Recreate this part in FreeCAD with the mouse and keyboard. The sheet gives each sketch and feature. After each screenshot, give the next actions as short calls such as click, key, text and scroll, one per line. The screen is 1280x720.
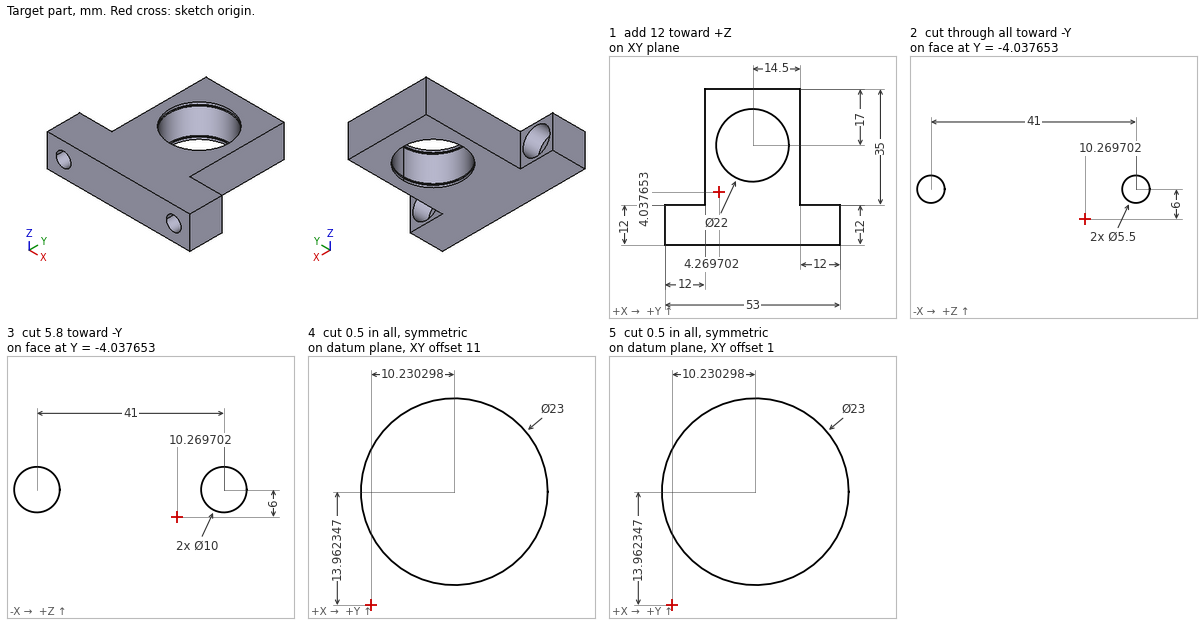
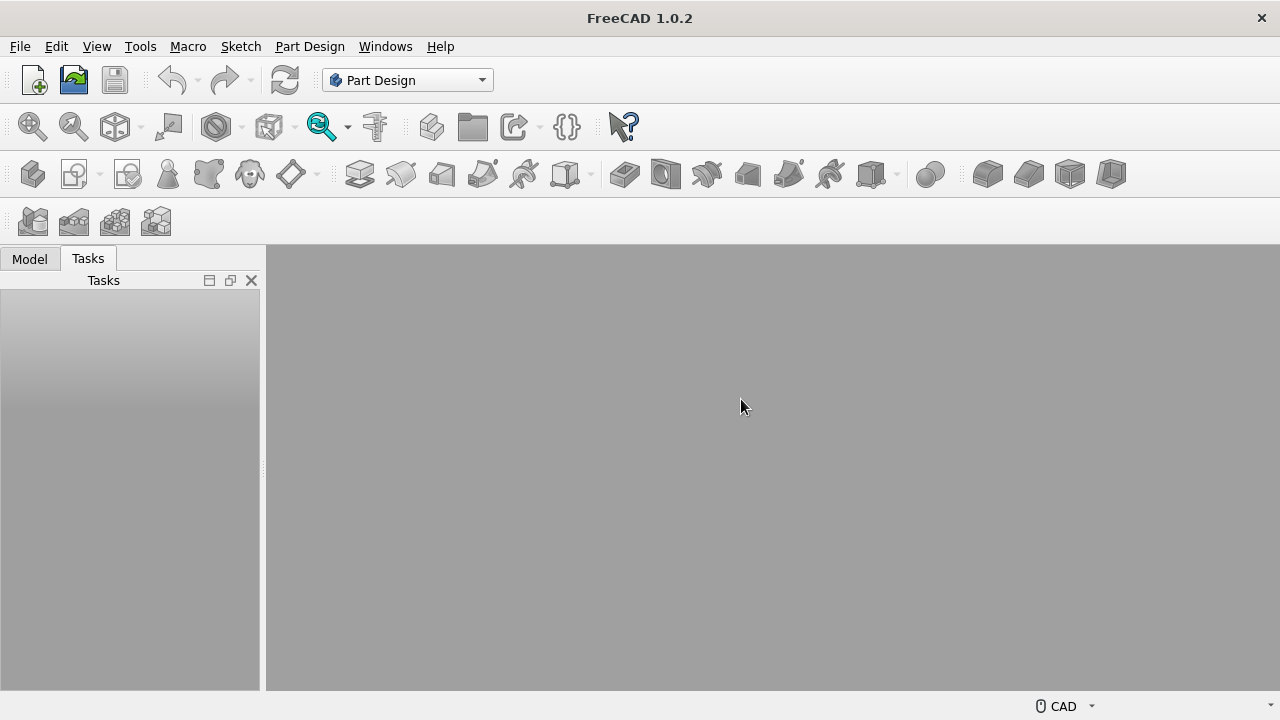
click(33, 80)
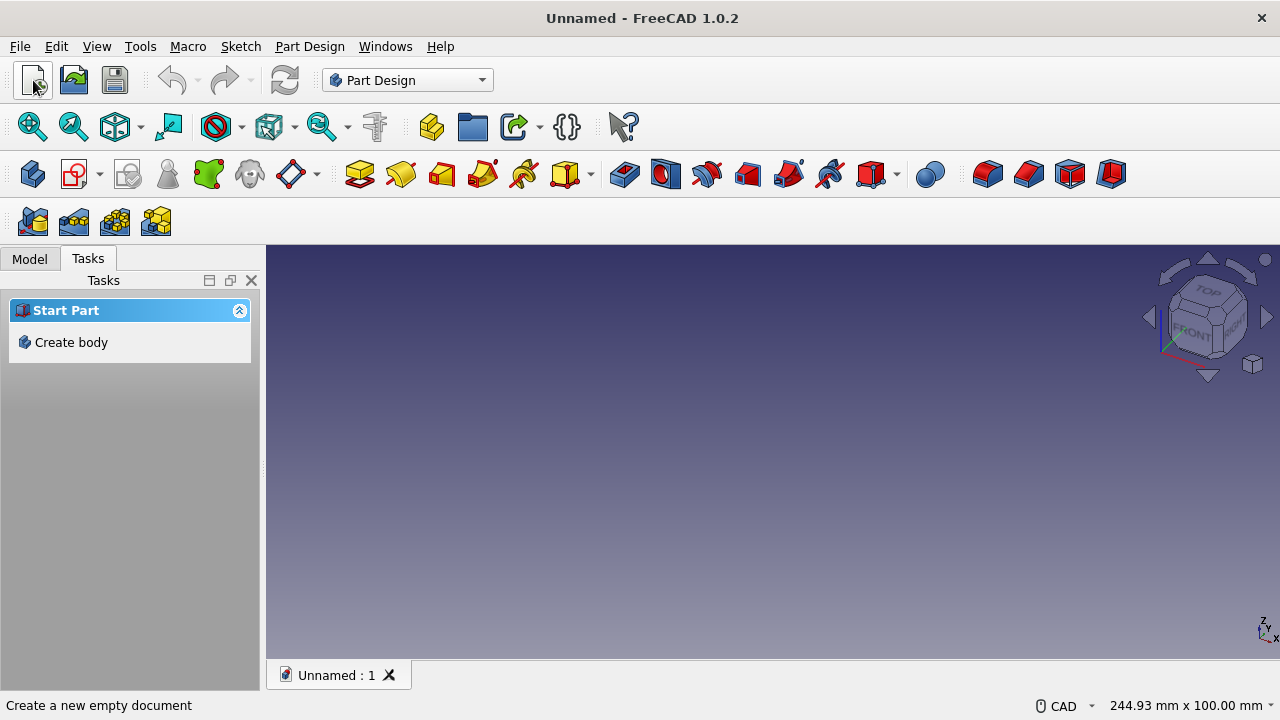
click(74, 174)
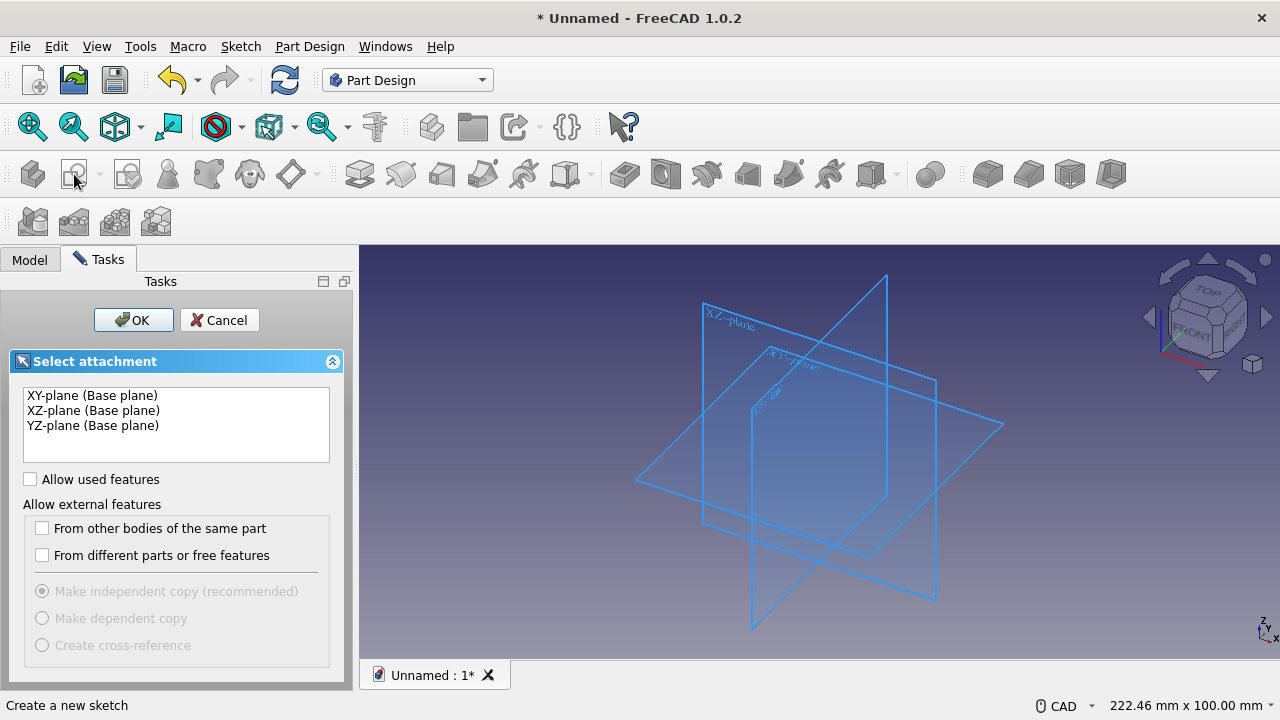
click(84, 396)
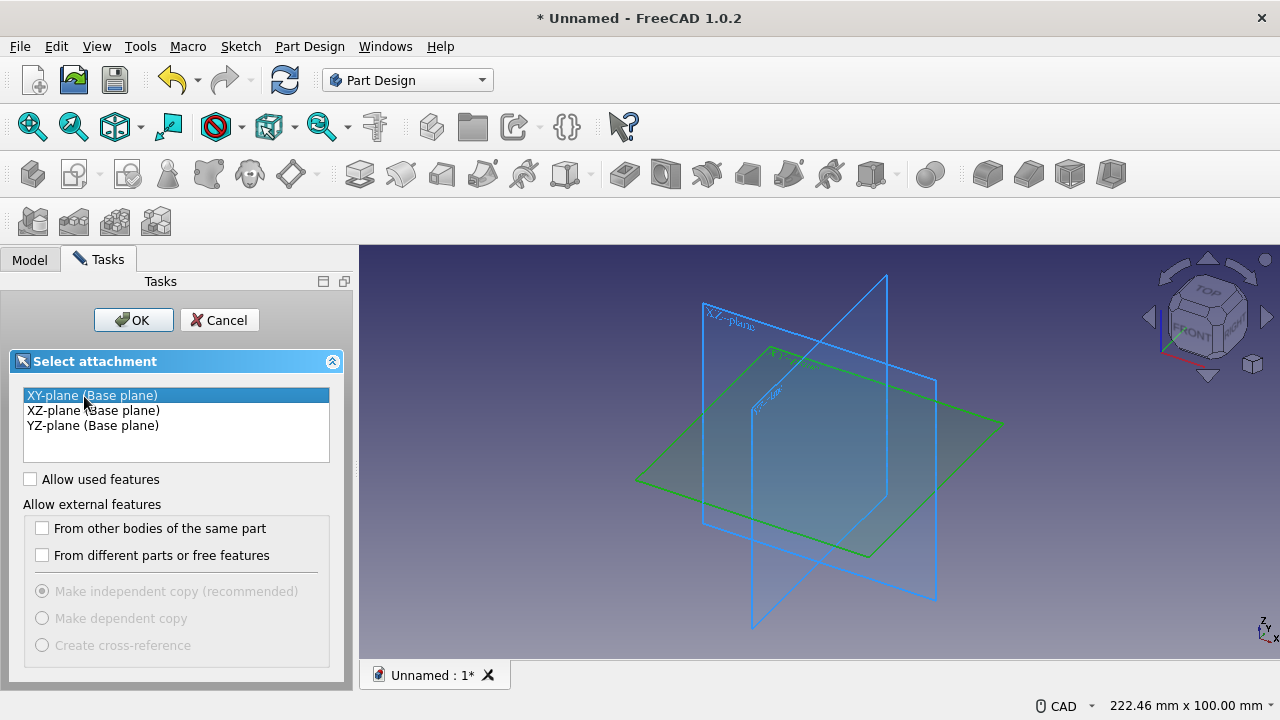
click(134, 320)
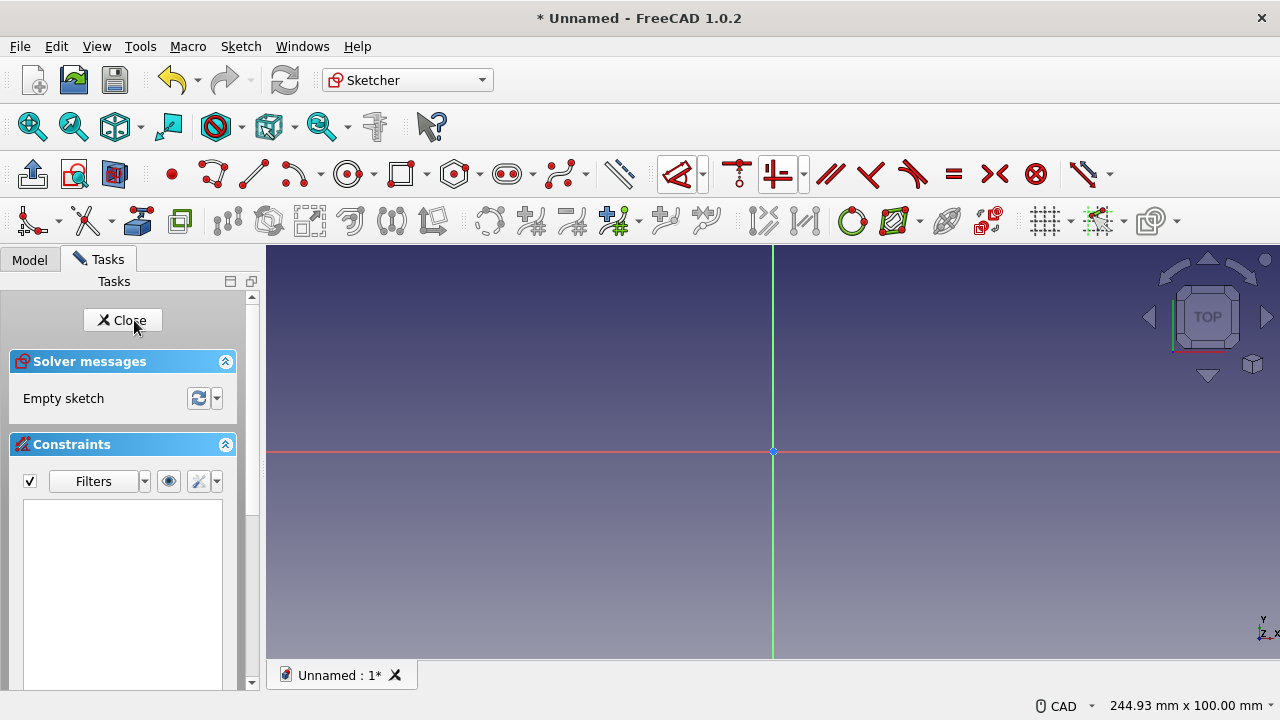
click(213, 174)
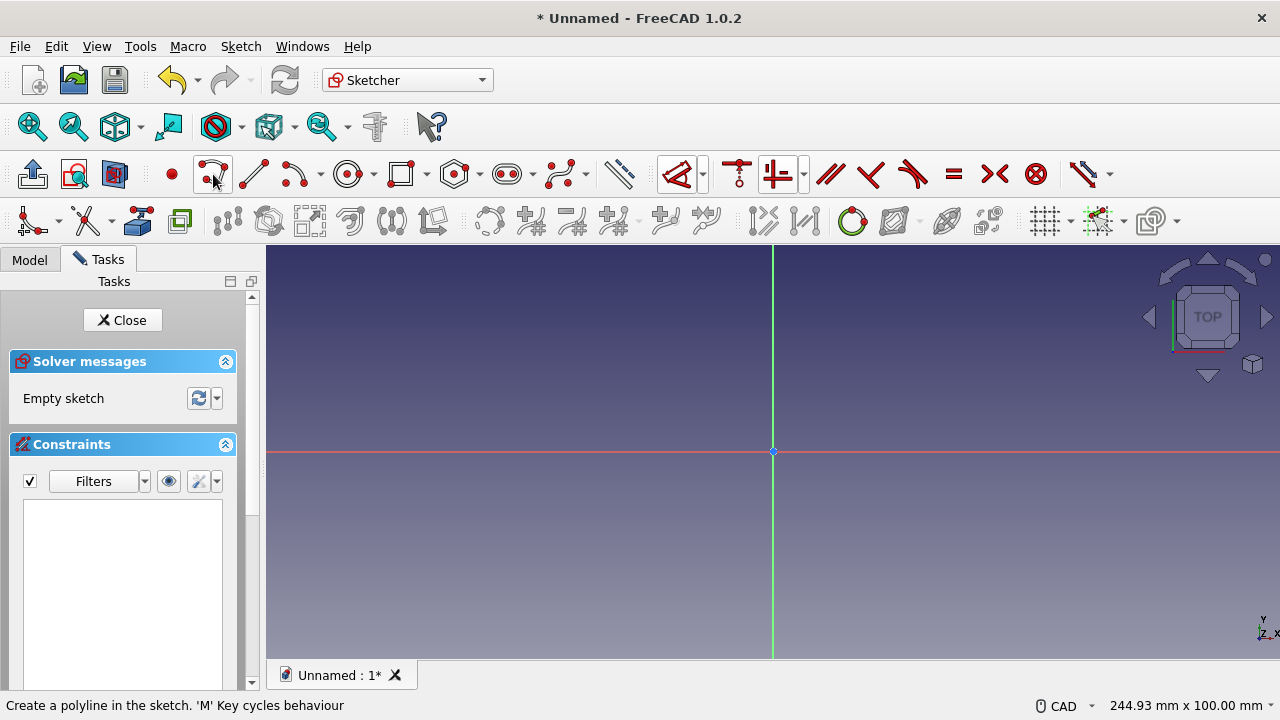
click(755, 469)
click(706, 469)
click(706, 518)
click(925, 518)
click(925, 469)
click(875, 469)
click(875, 324)
click(755, 324)
click(755, 470)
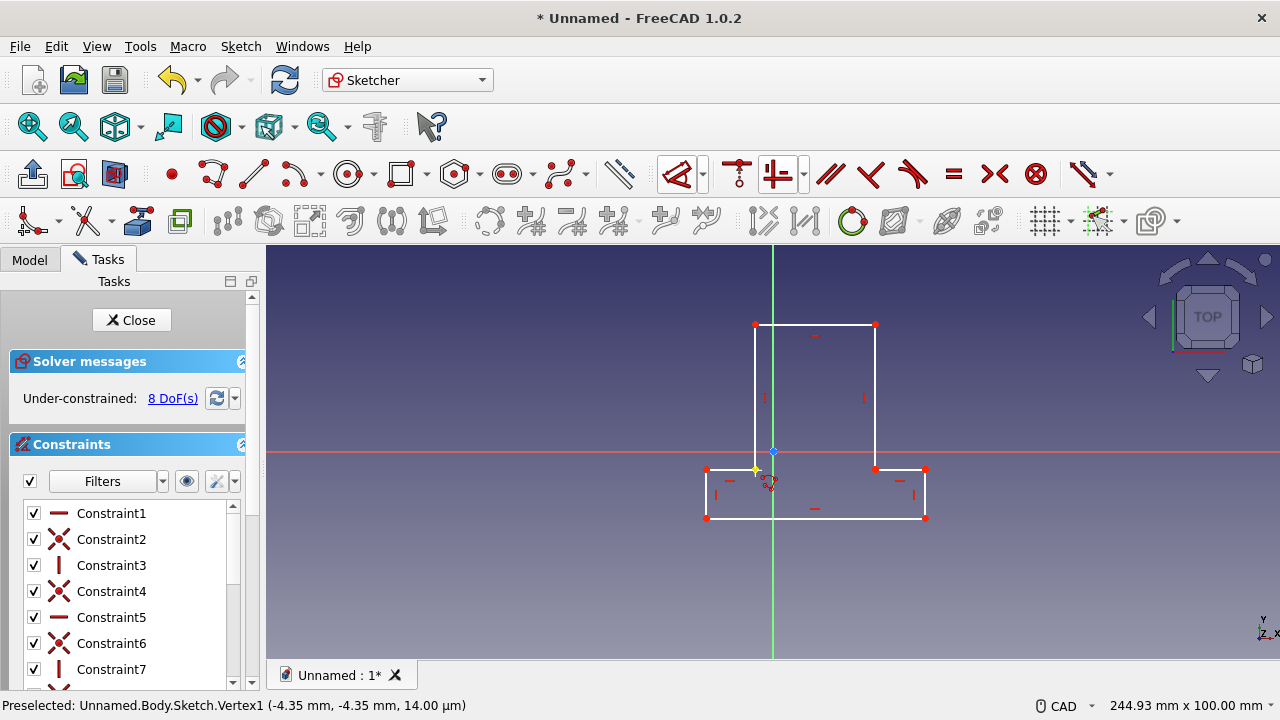
click(348, 174)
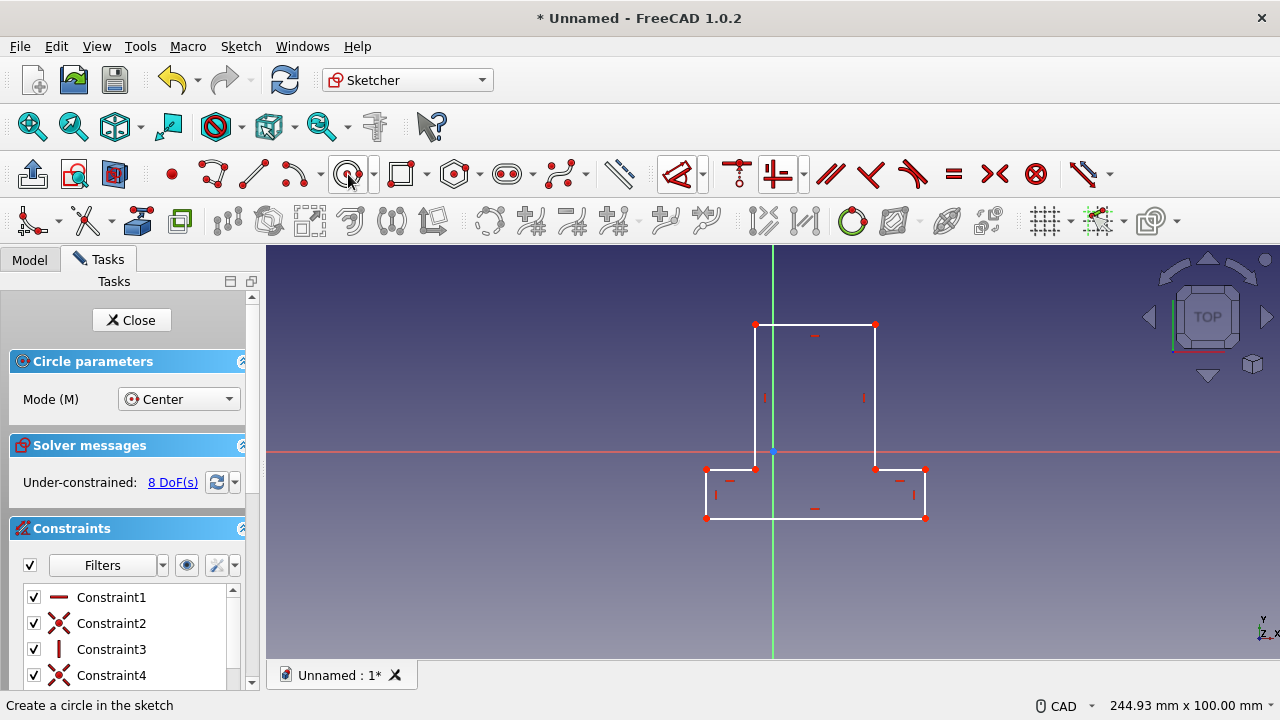
click(815, 394)
click(848, 362)
key(Escape)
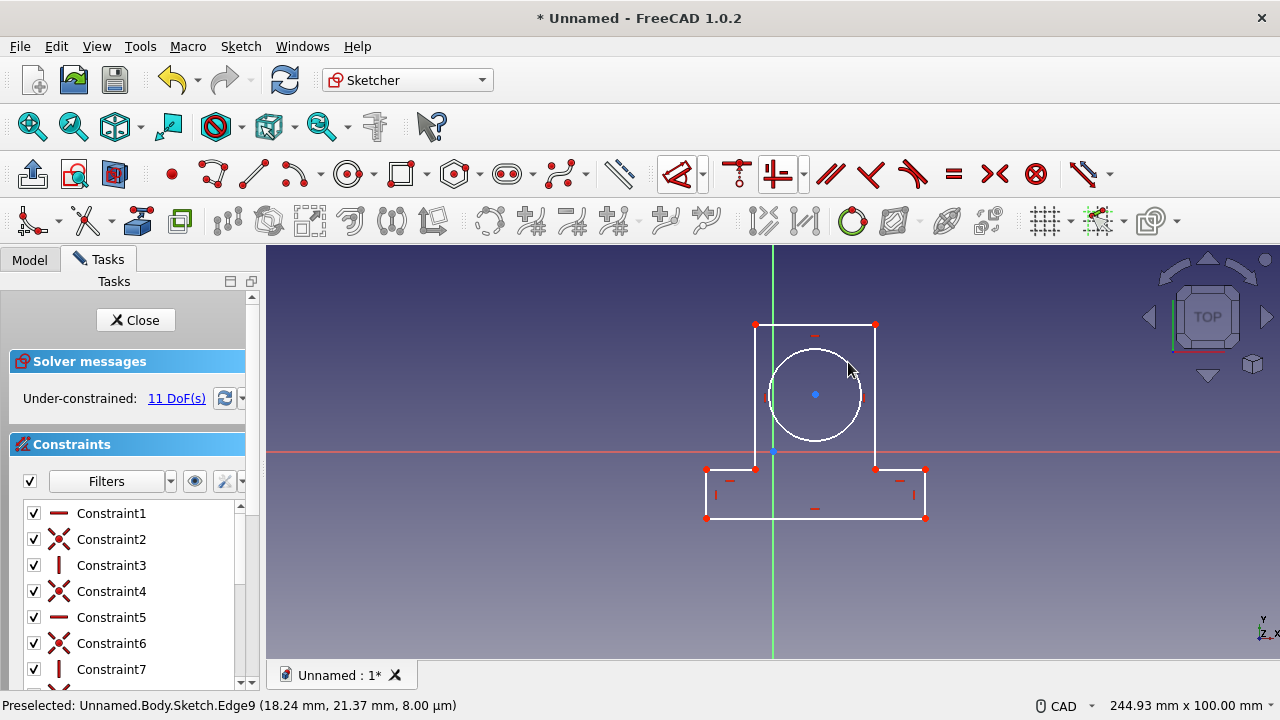
click(676, 174)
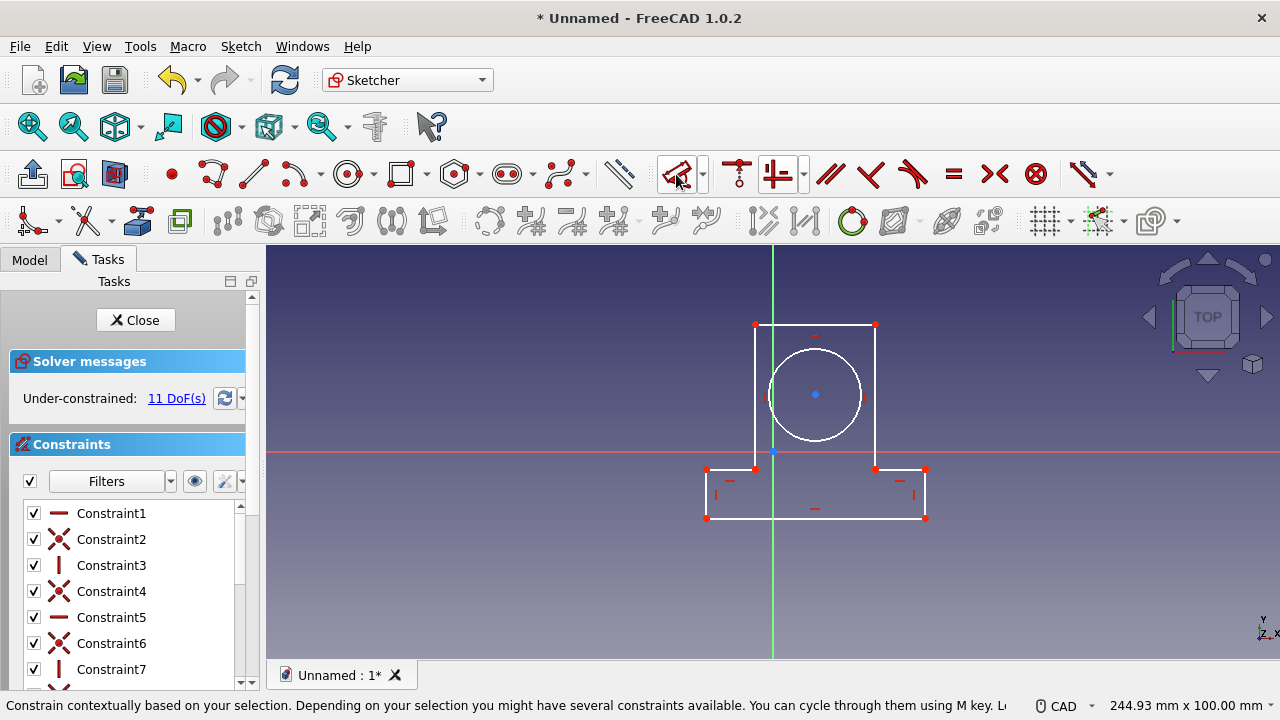
click(847, 362)
click(889, 372)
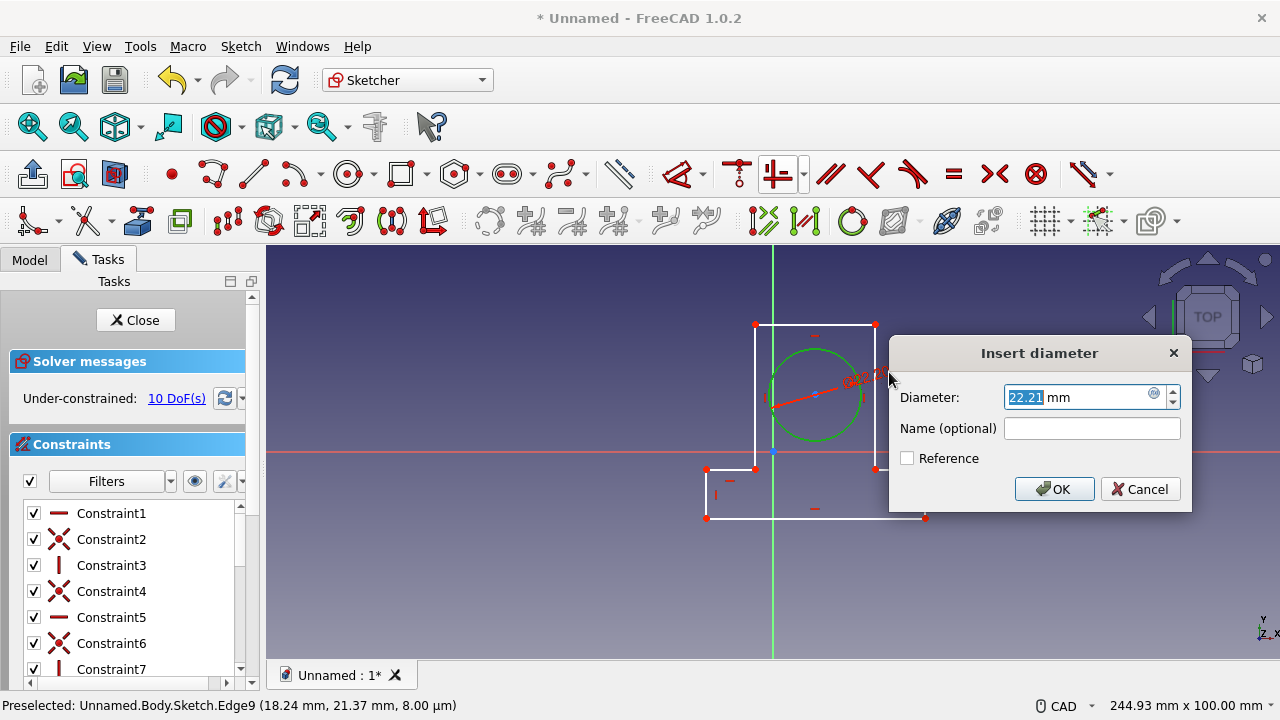
text(22)
key(Return)